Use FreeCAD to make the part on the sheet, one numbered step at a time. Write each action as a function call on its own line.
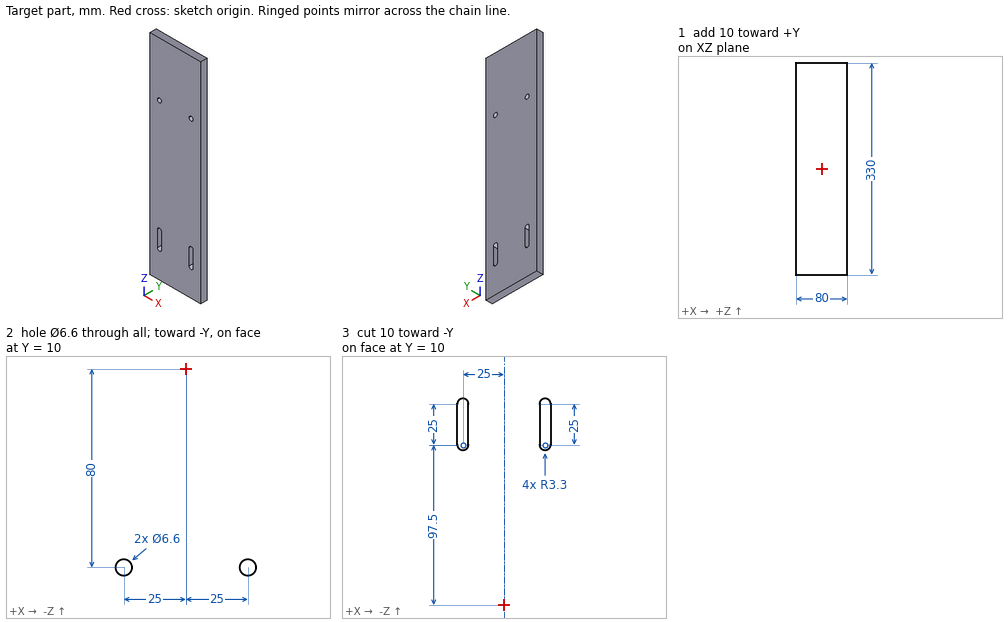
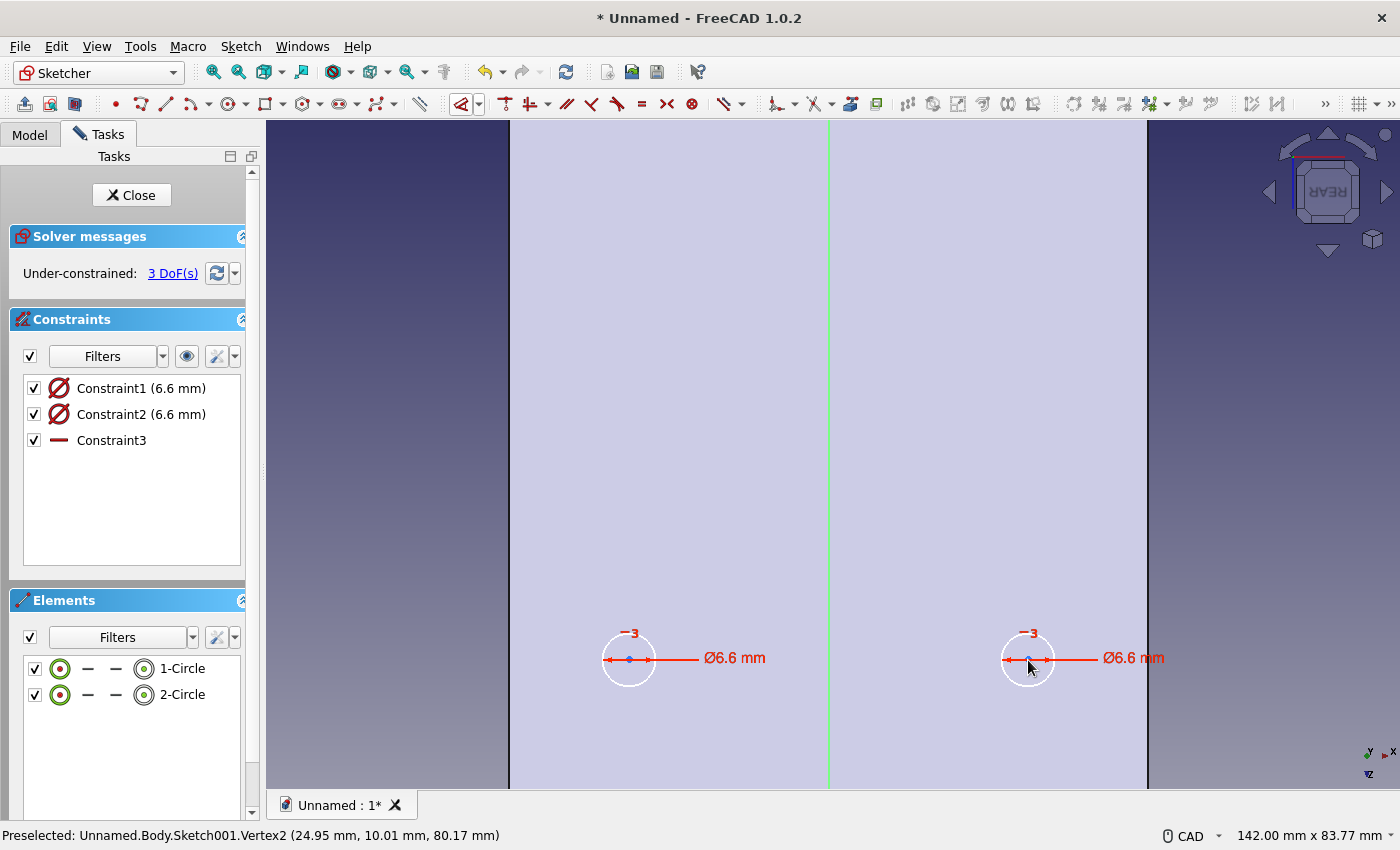
click(460, 104)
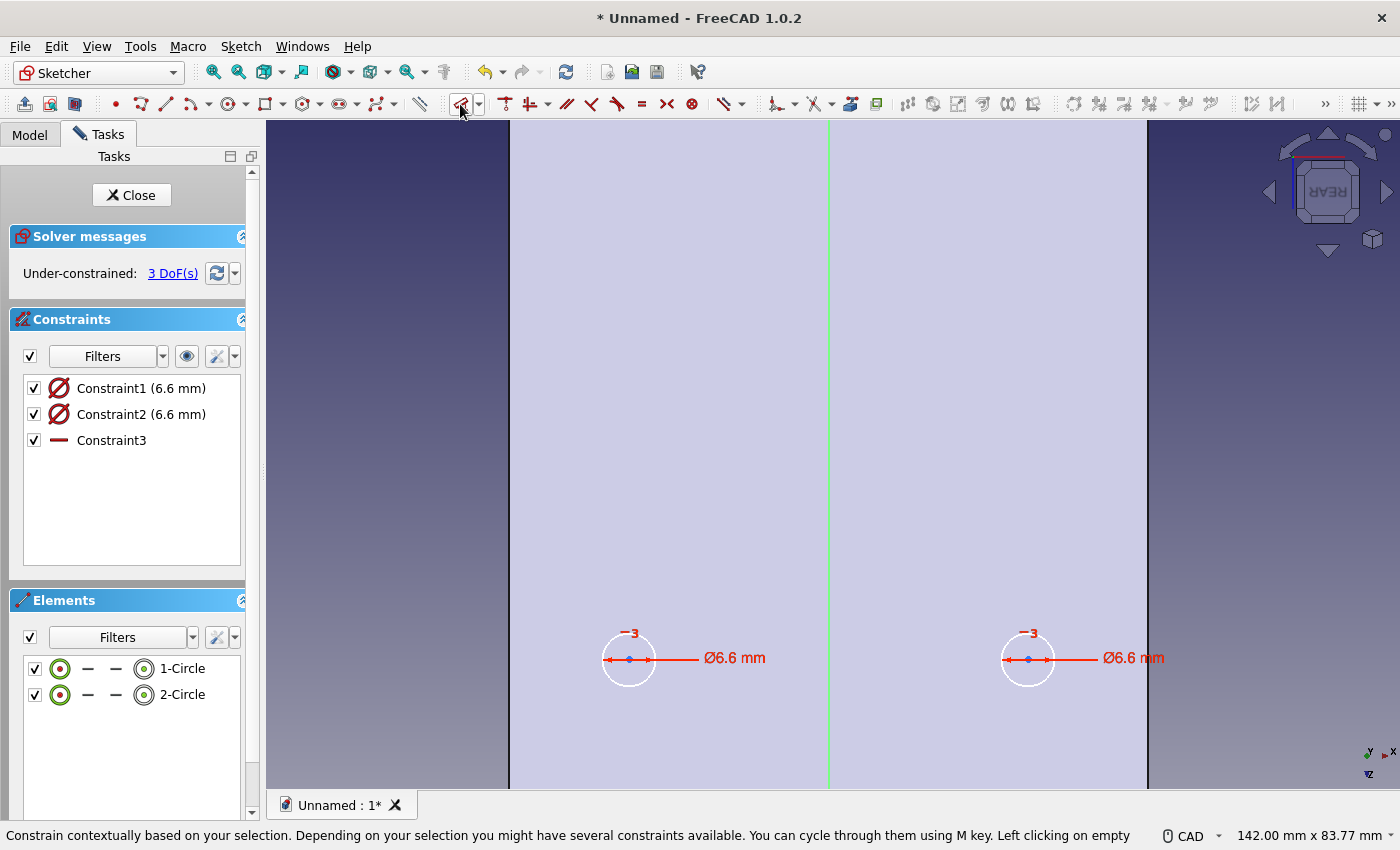
click(629, 660)
click(729, 694)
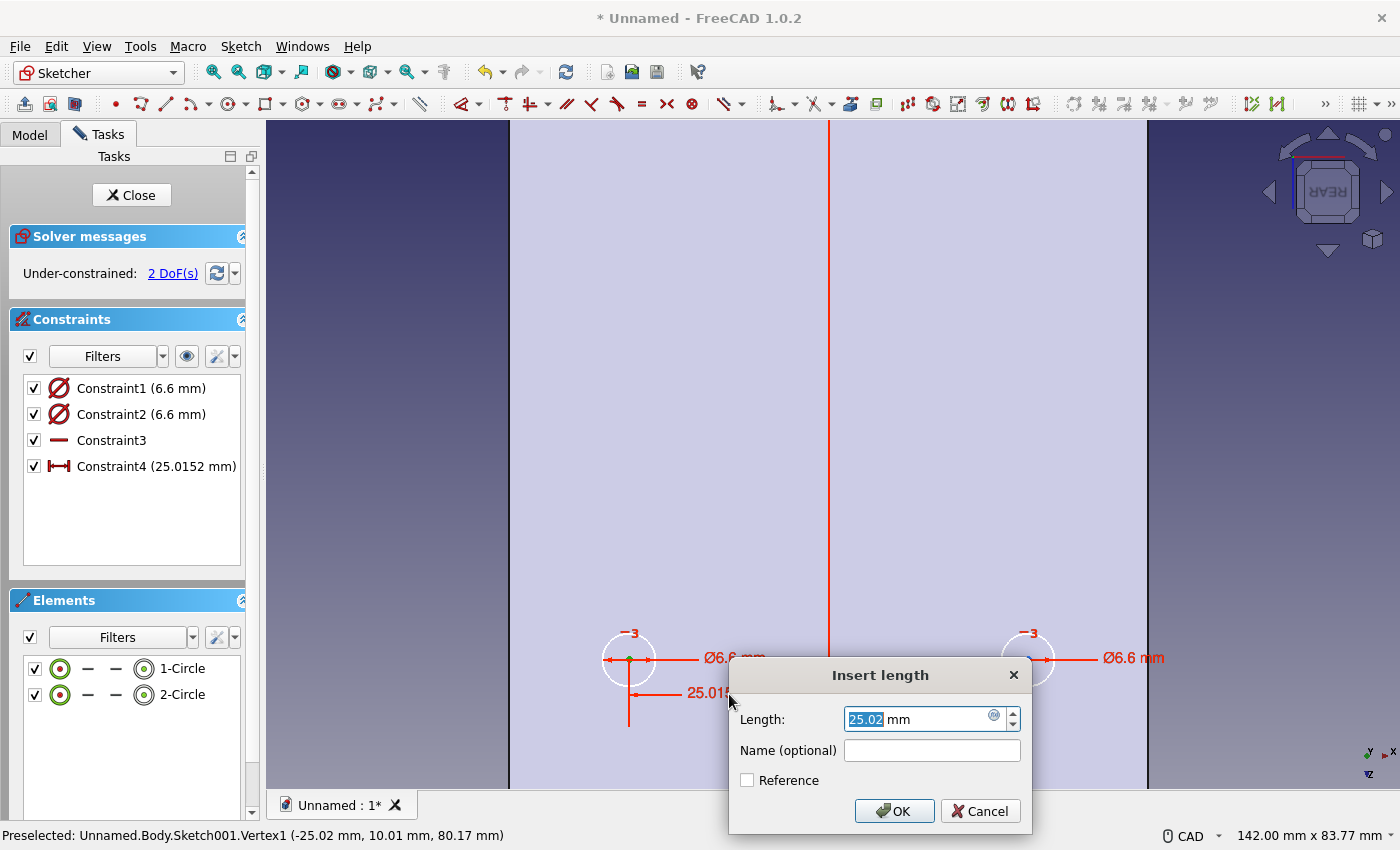
text(25)
key(Return)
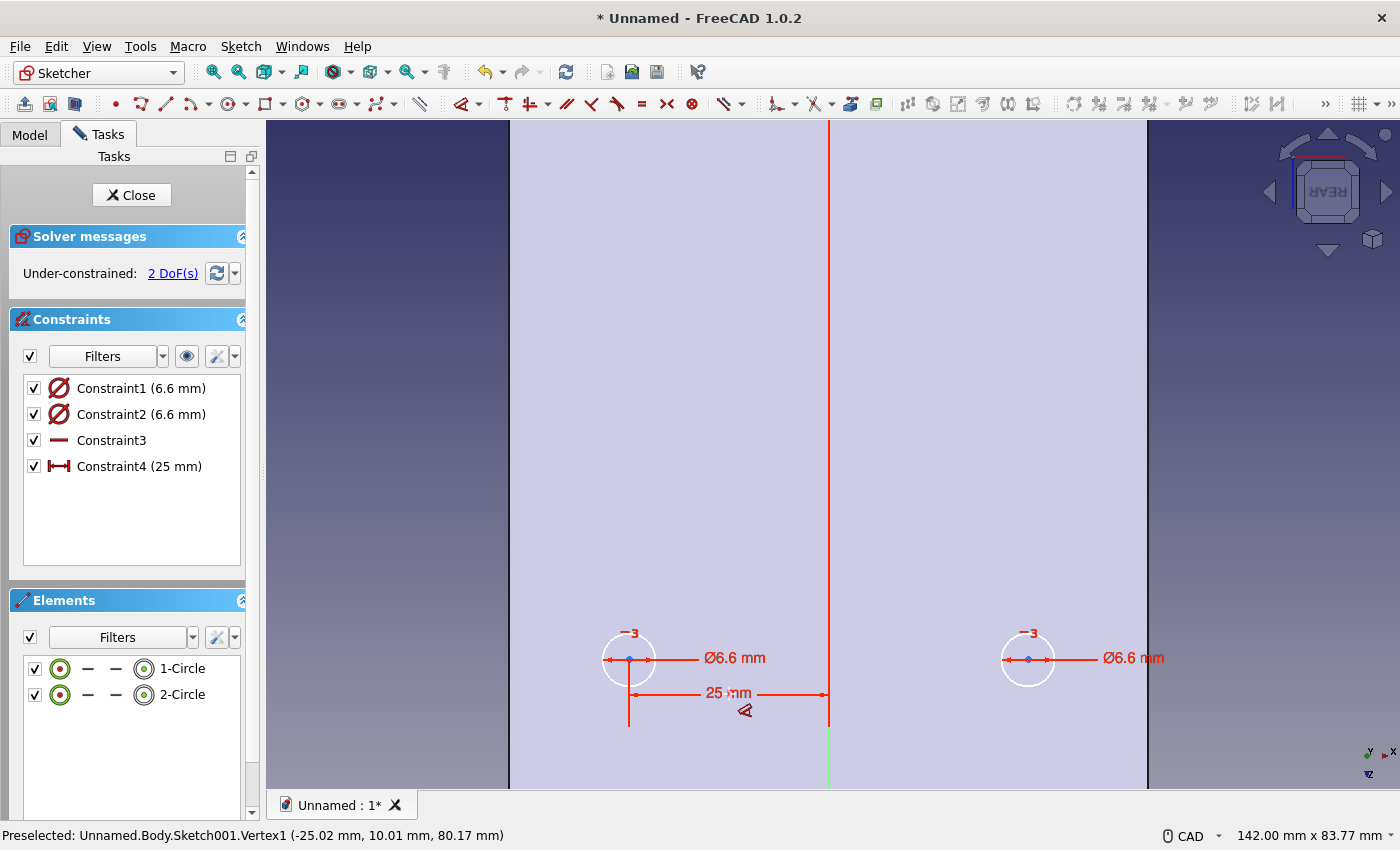
click(629, 660)
click(595, 404)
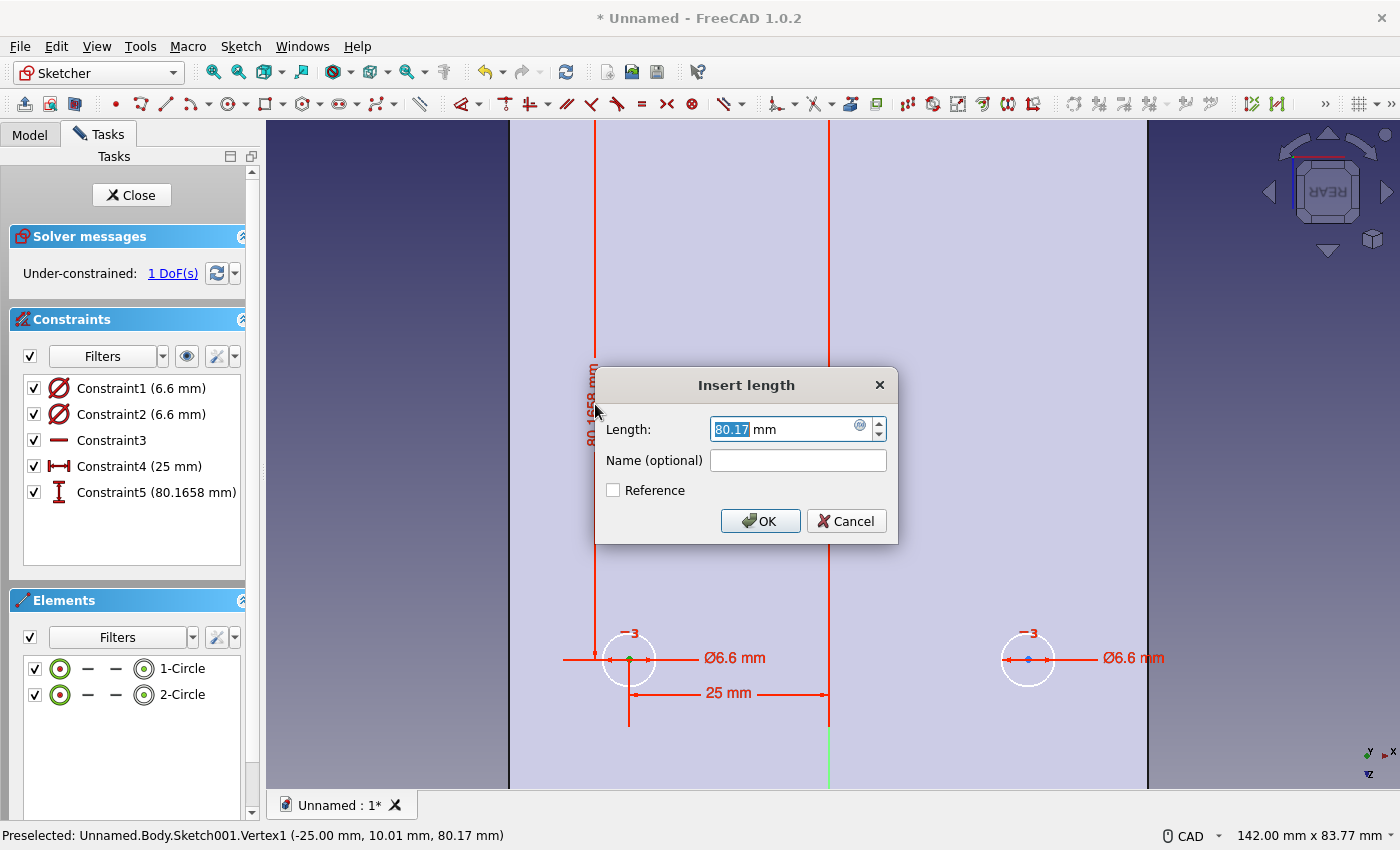
text(80)
key(Return)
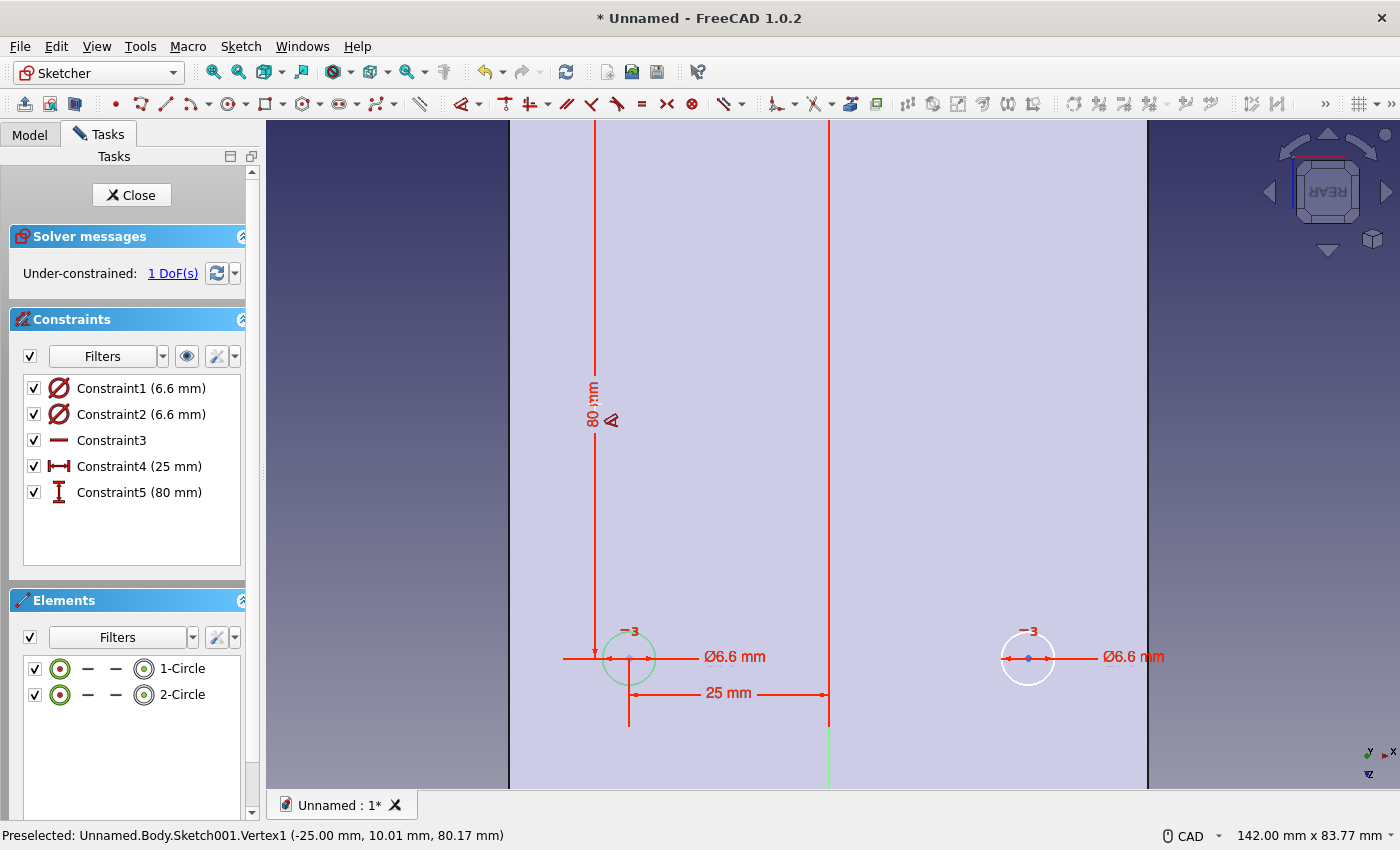
click(1028, 659)
click(928, 693)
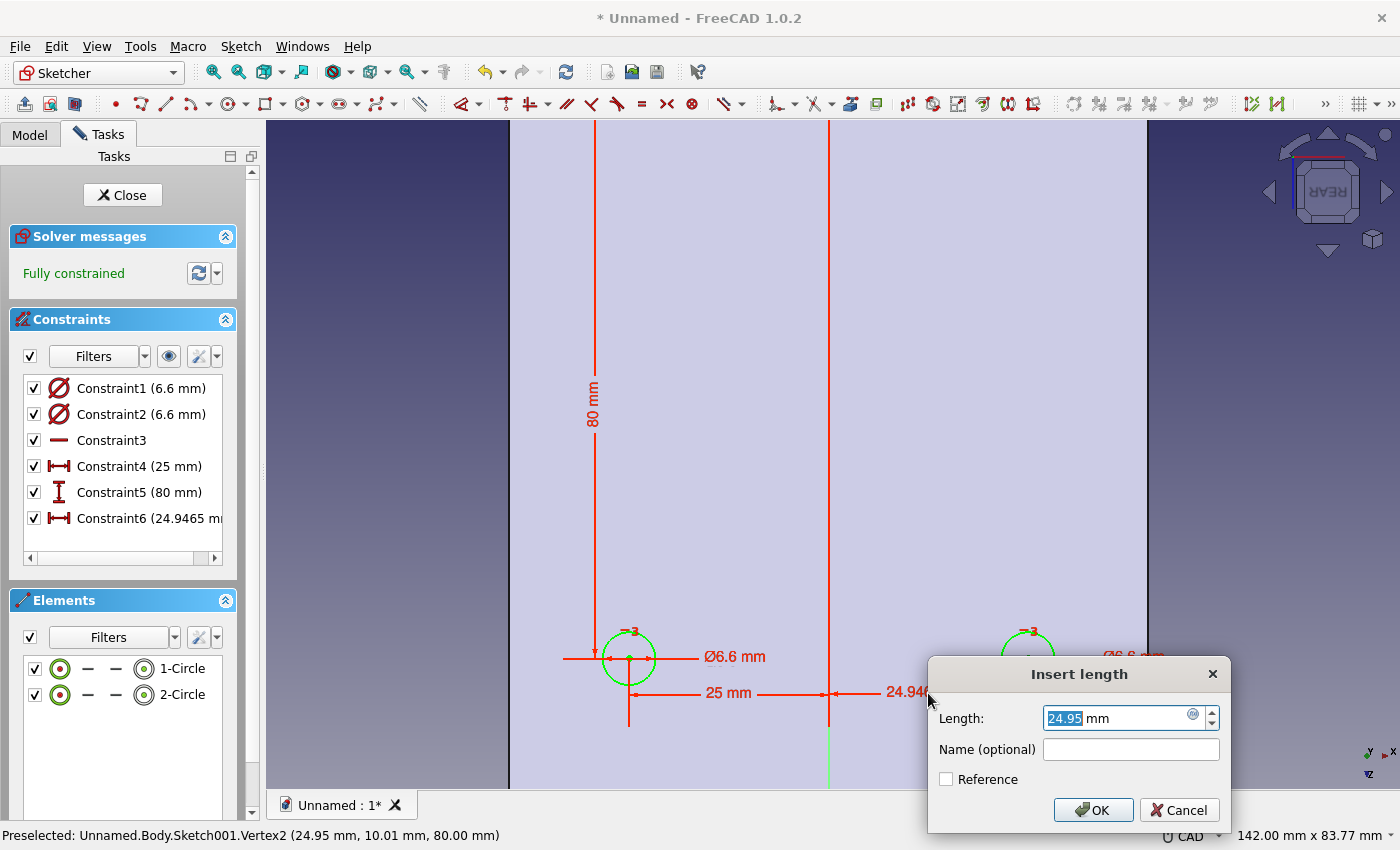
text(25)
key(Return)
key(Escape)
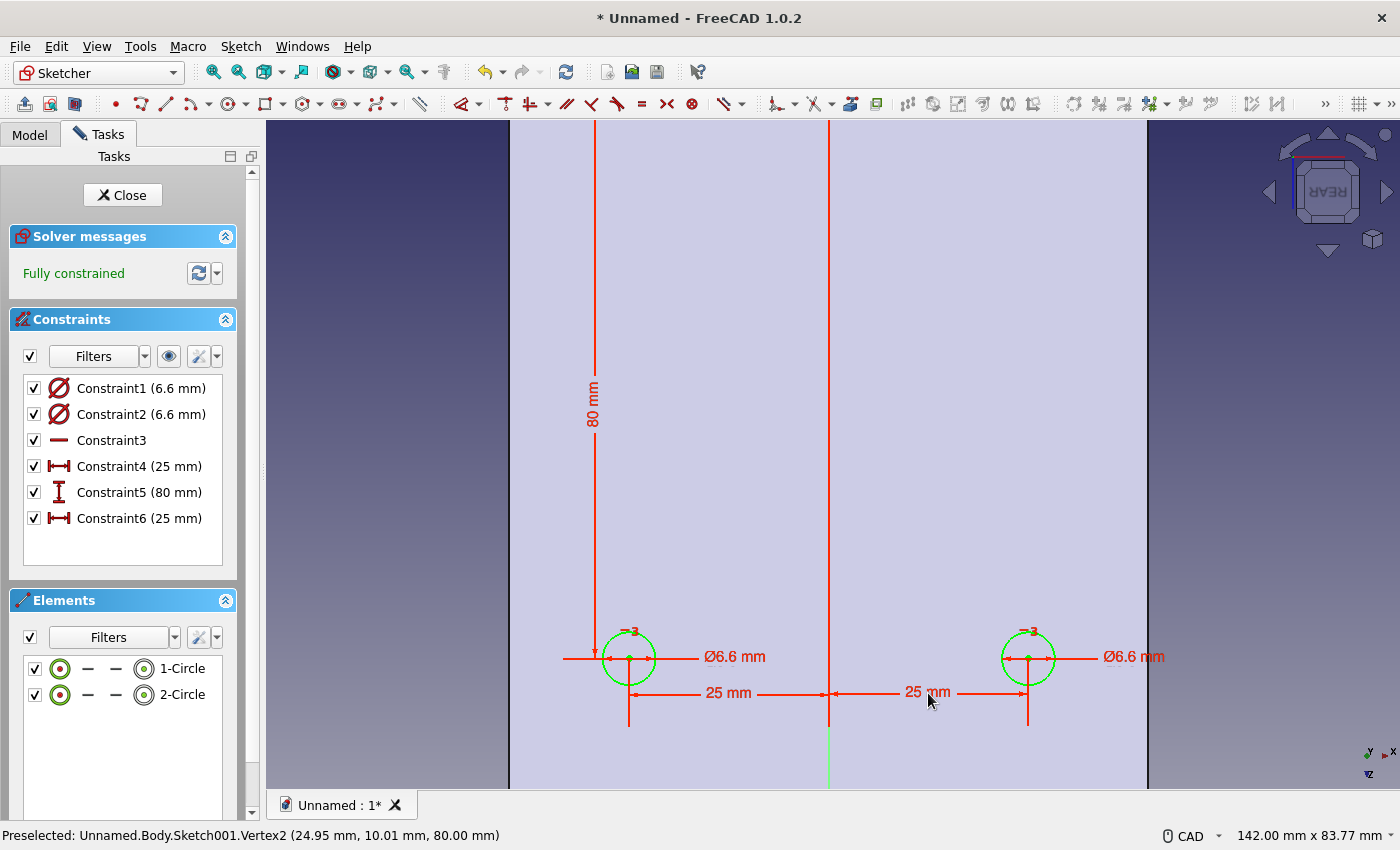
click(123, 195)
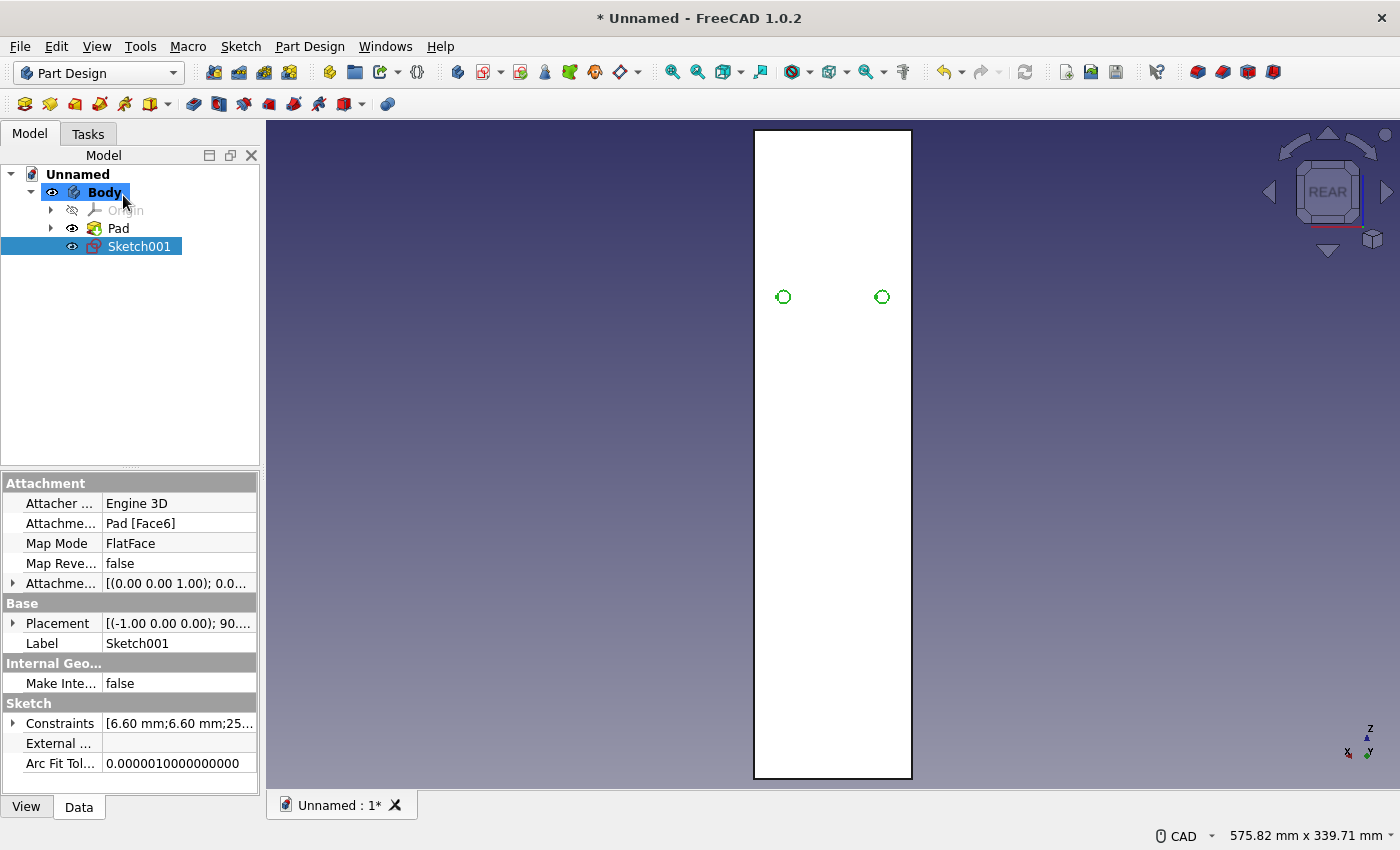
click(219, 104)